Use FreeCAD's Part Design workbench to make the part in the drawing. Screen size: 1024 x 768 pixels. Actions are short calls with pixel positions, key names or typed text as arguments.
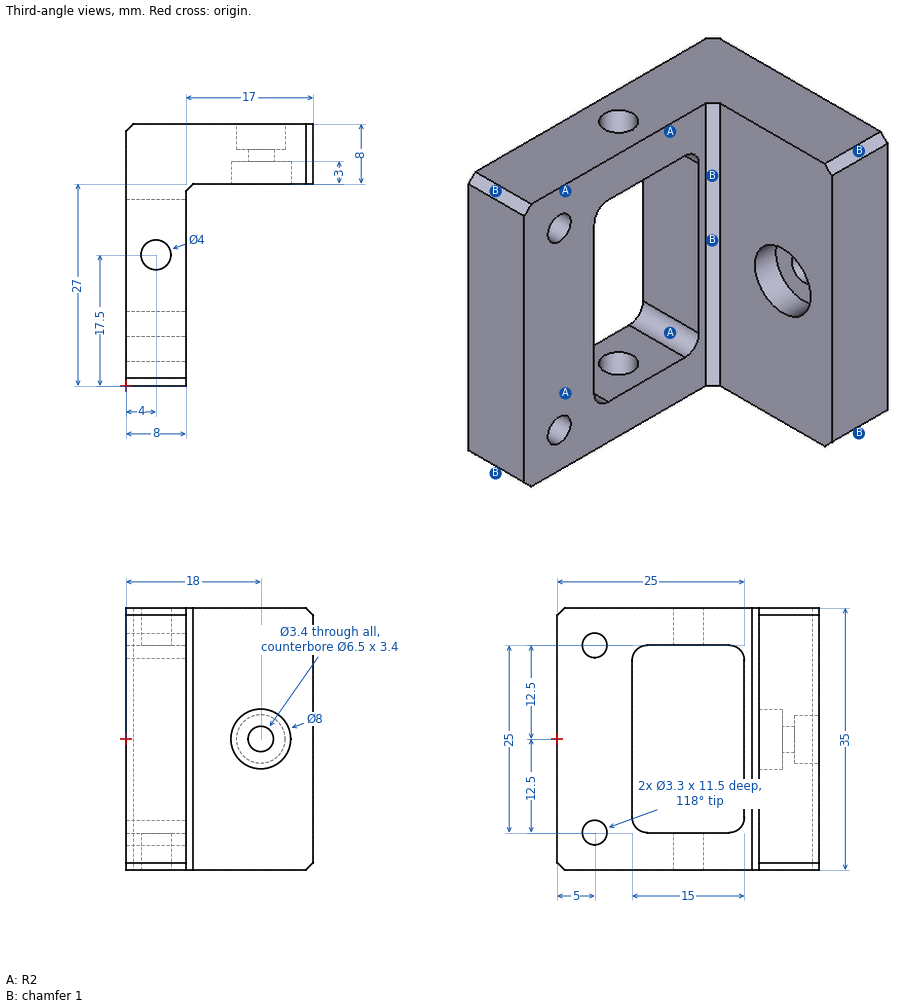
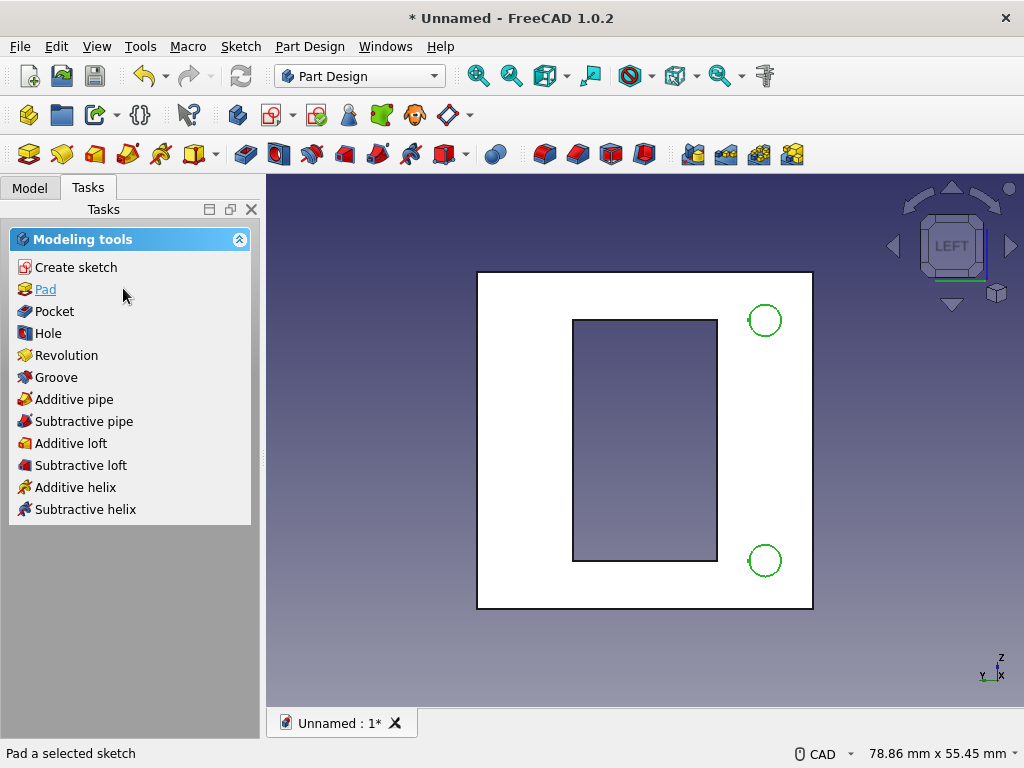
click(279, 154)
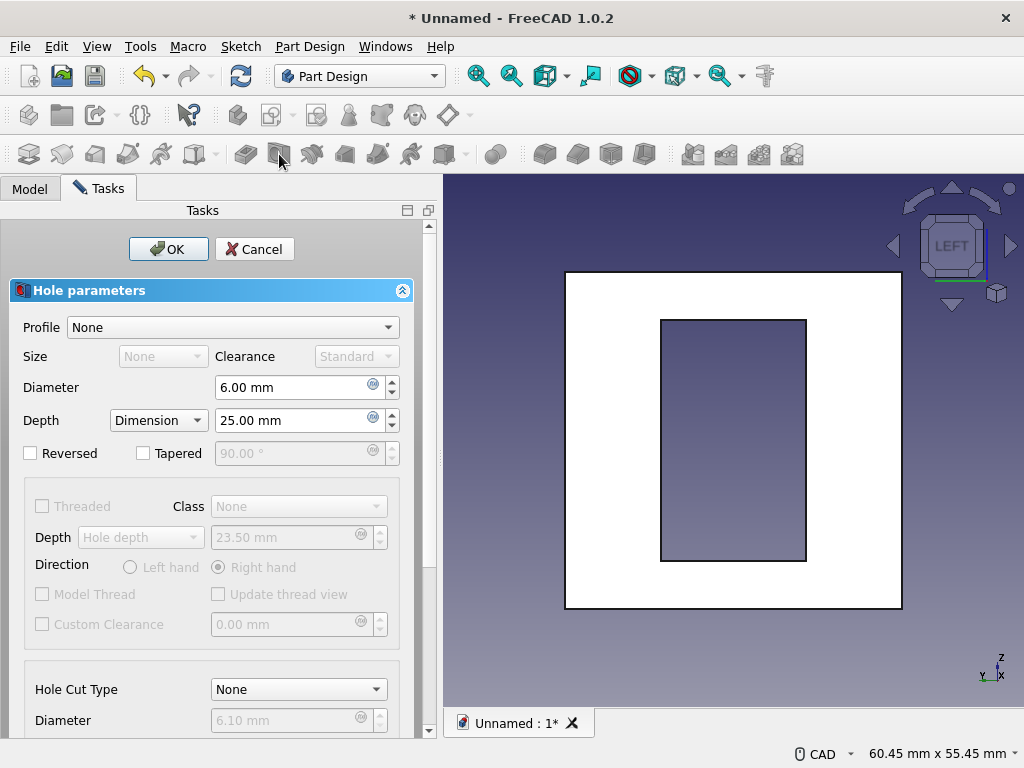
triple_click(300, 388)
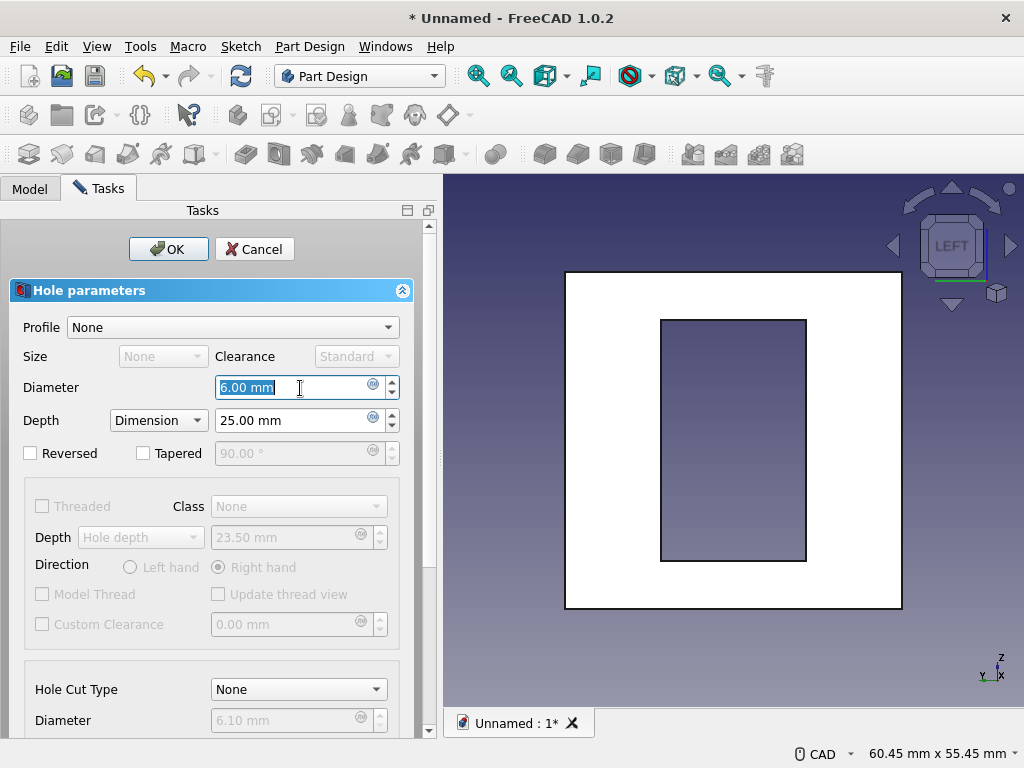
text(3.3)
key(Tab)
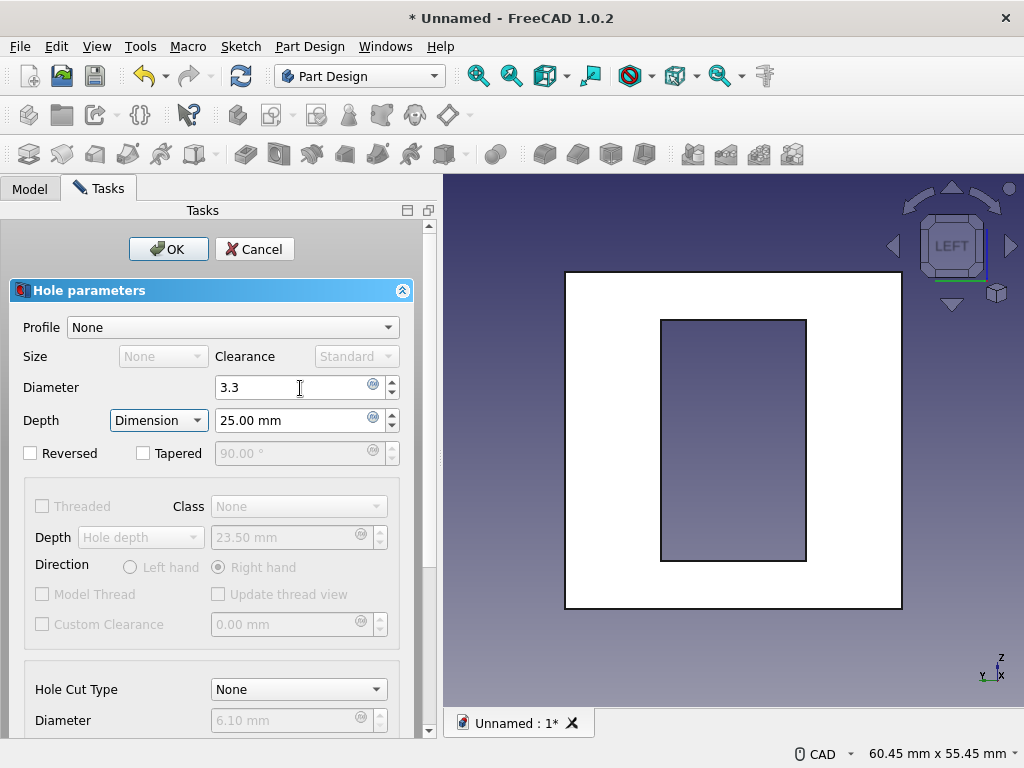
triple_click(300, 420)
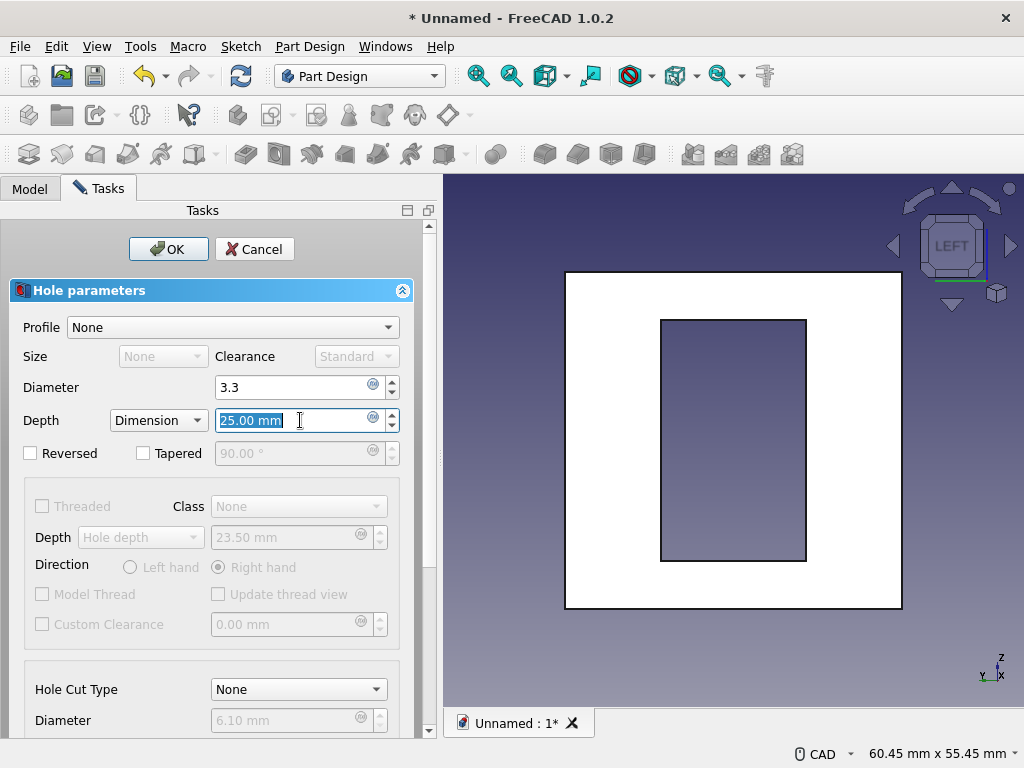
text(11.5)
key(Tab)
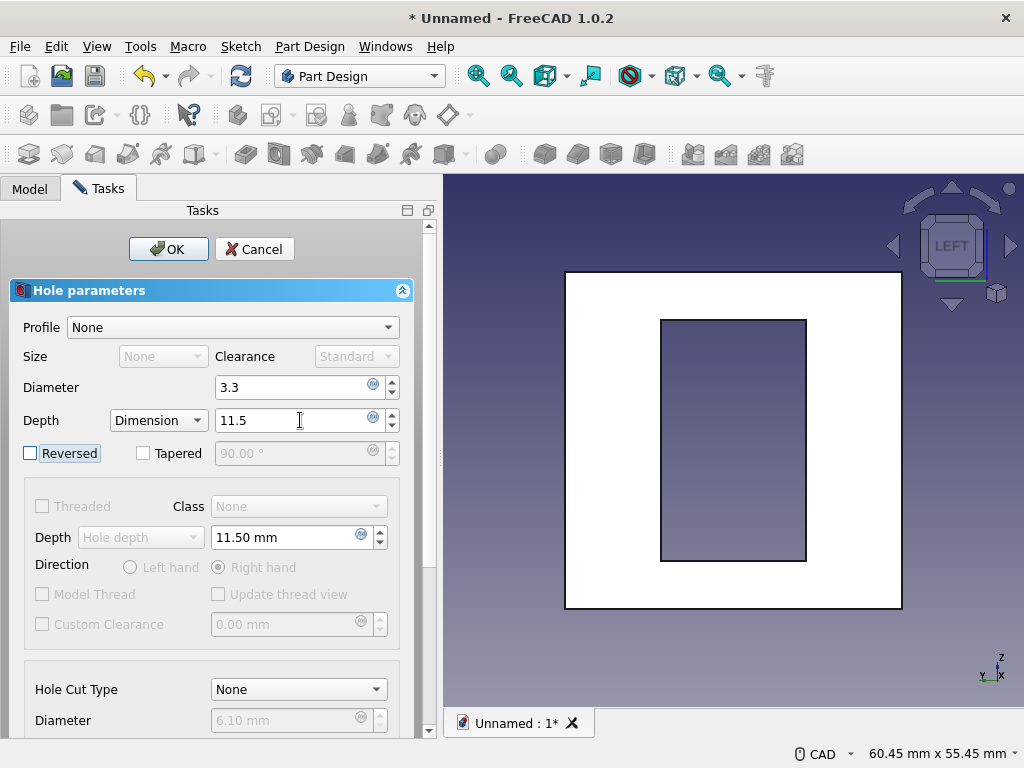
click(31, 453)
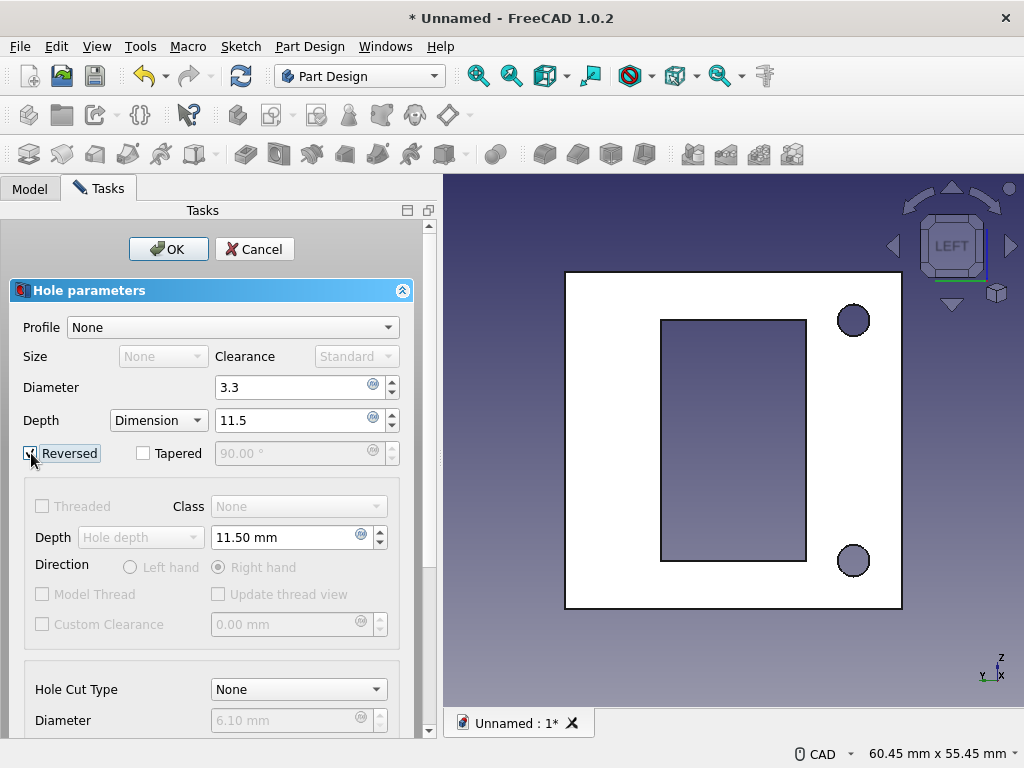
click(169, 249)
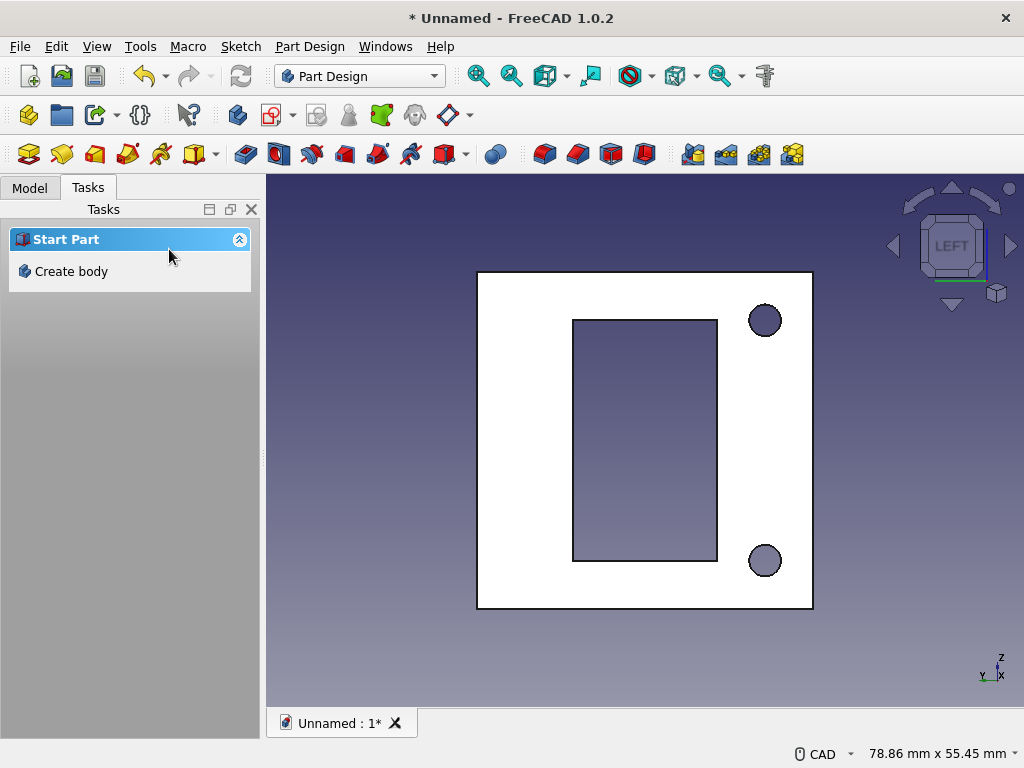
key(0)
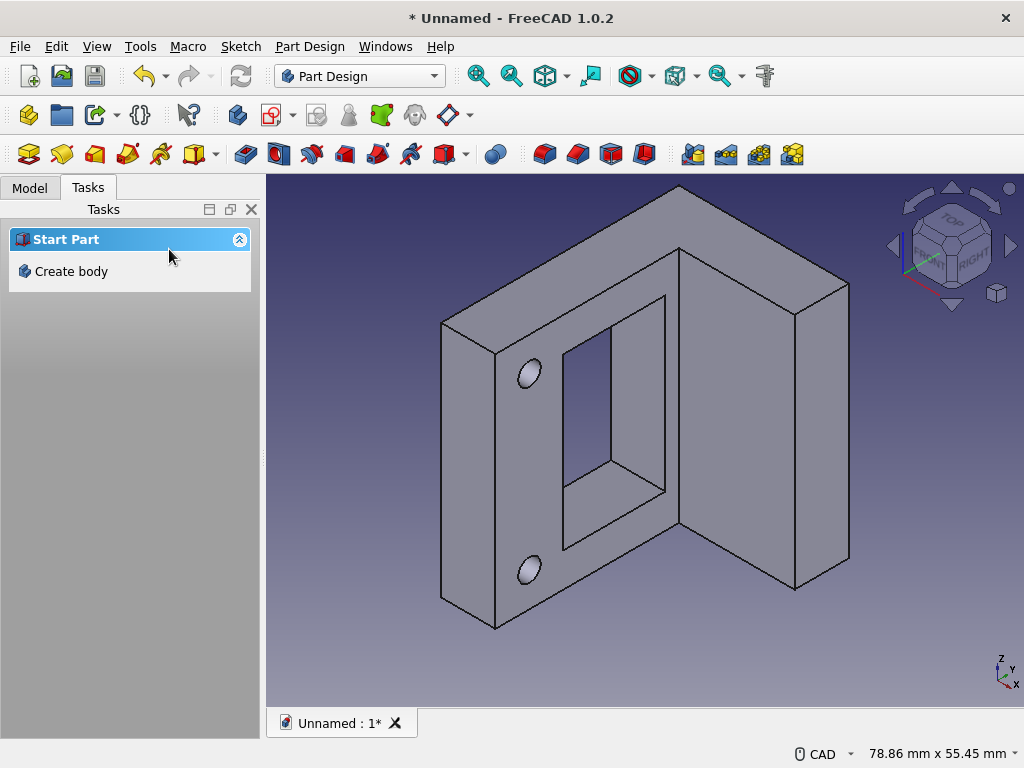
click(664, 235)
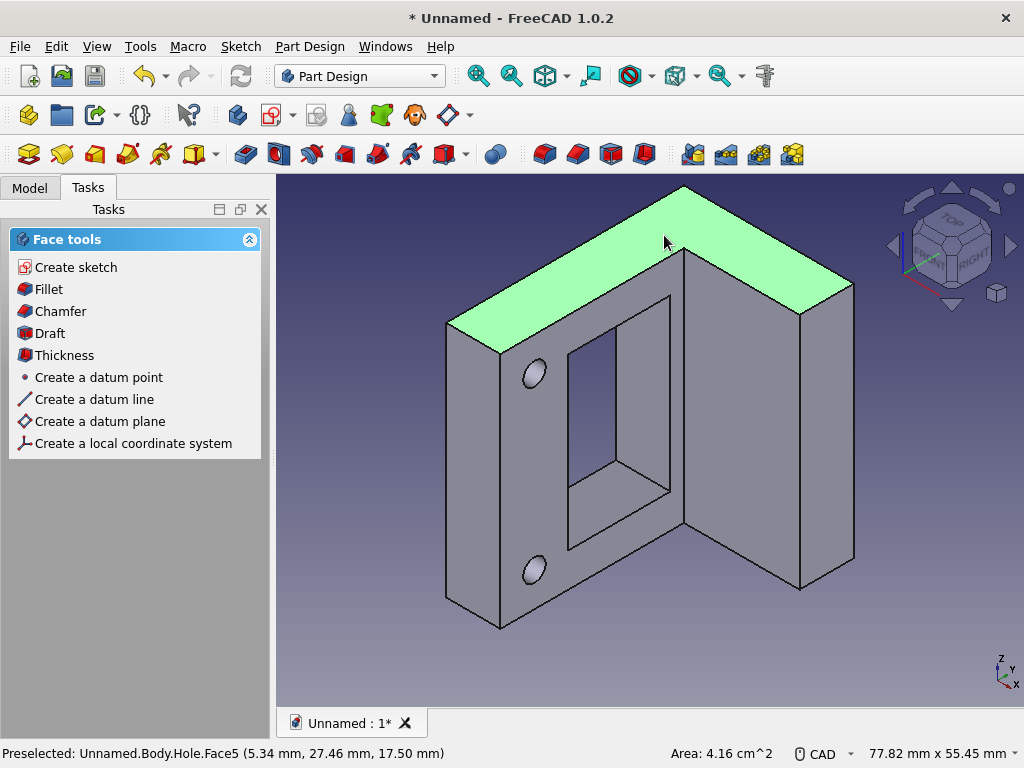
click(270, 116)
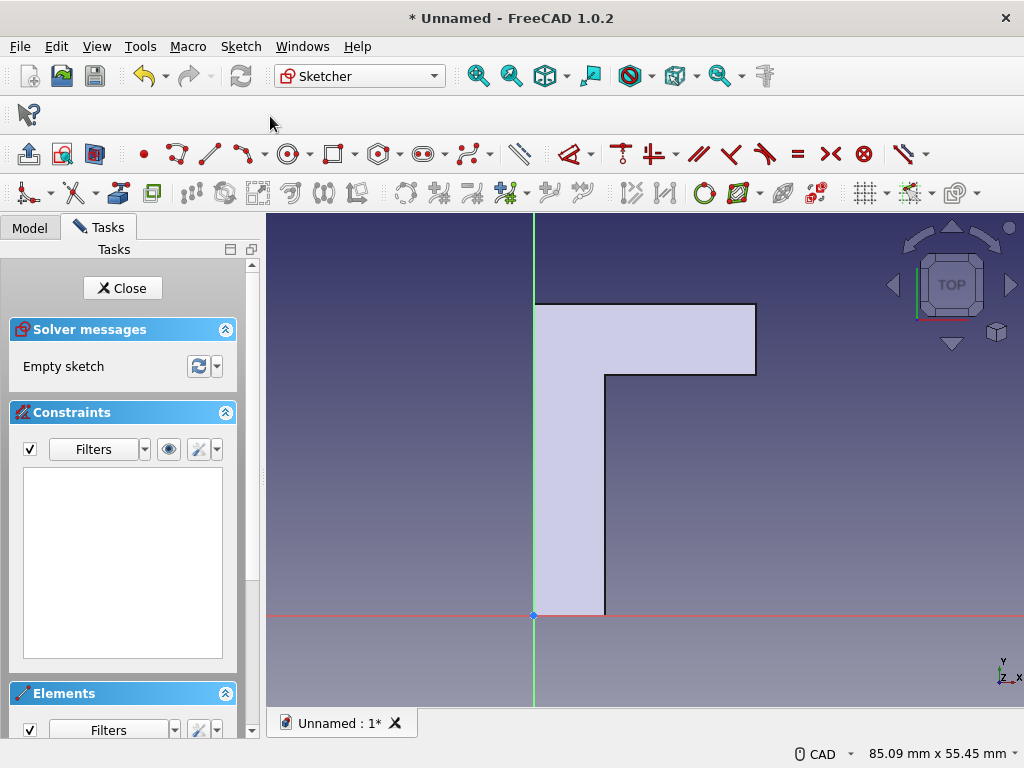
scroll(568, 460, up, 11)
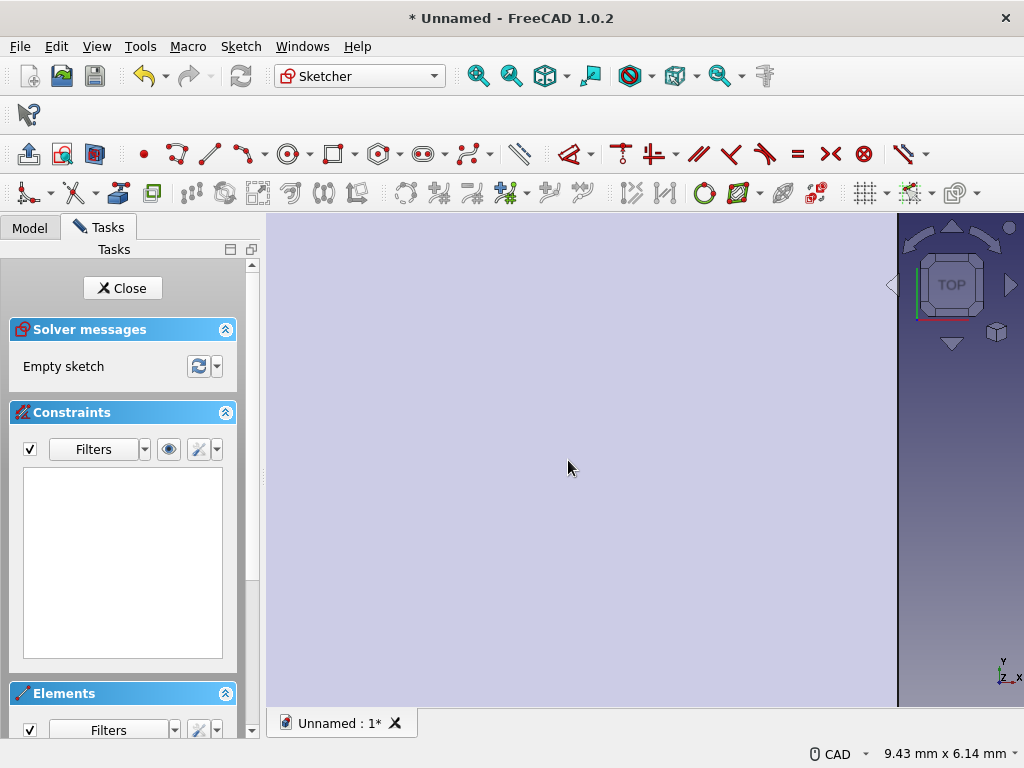
key(g)
key(c)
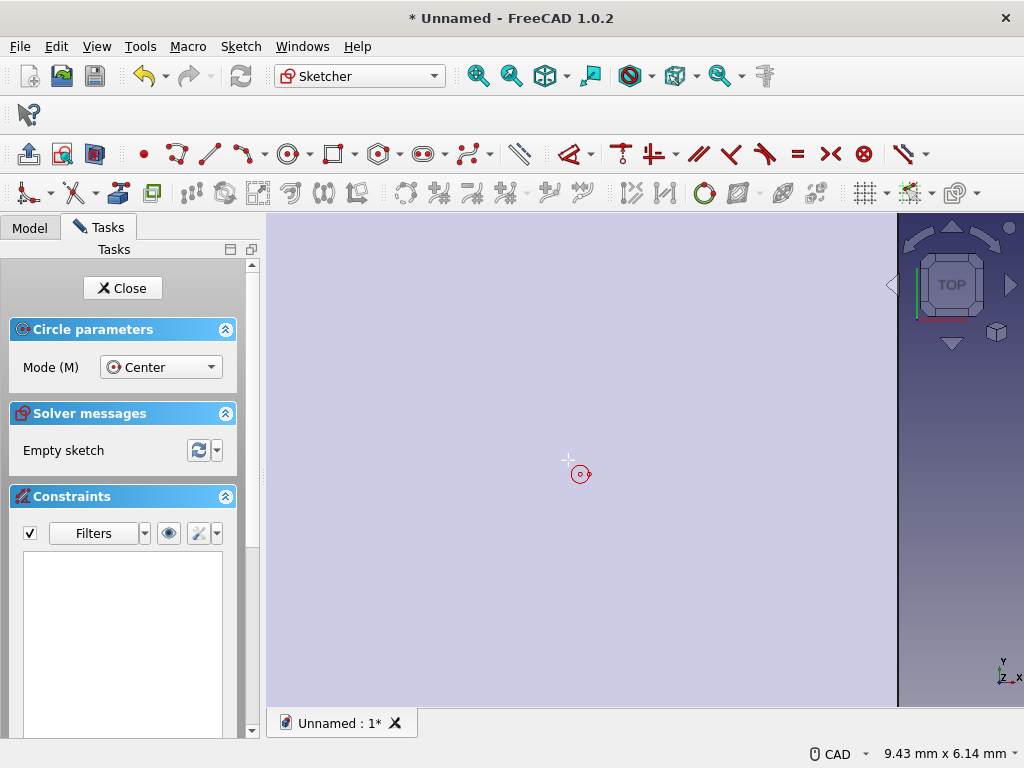
click(576, 456)
move(690, 342)